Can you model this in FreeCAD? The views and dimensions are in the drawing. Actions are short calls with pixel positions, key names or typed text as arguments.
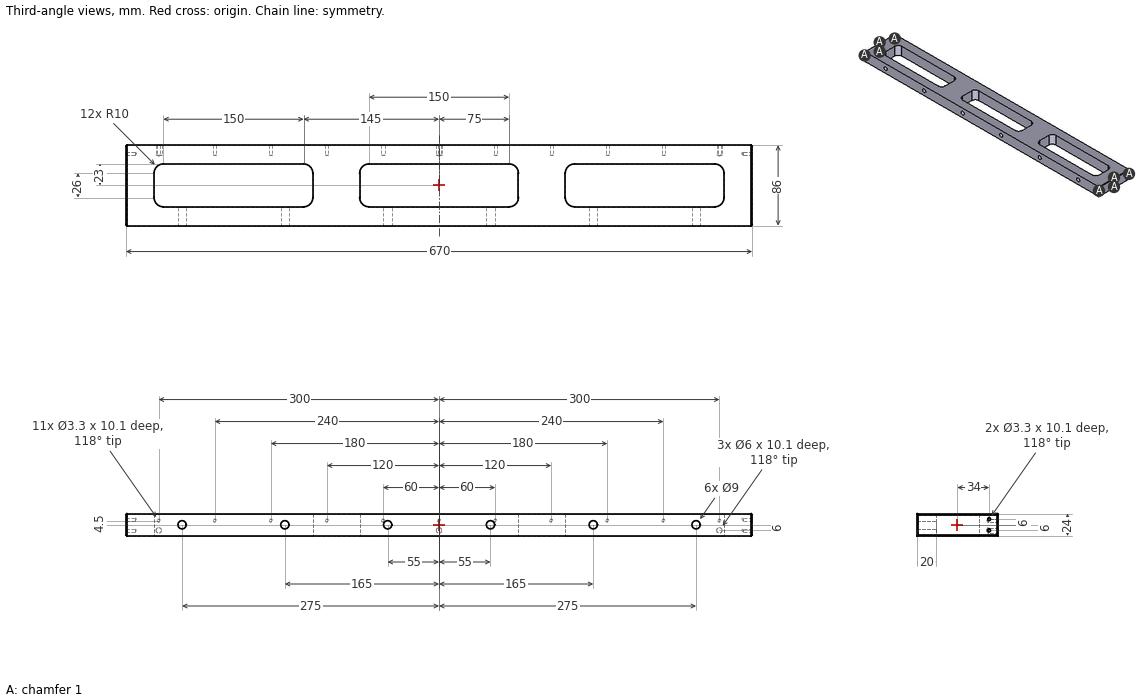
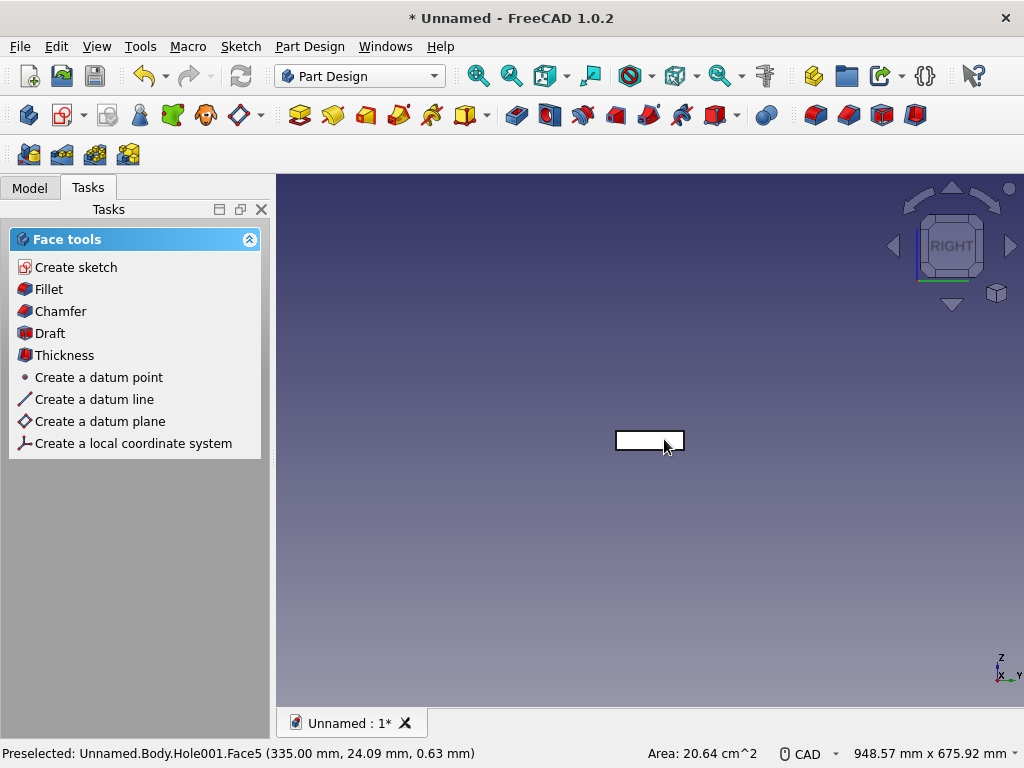
key(5)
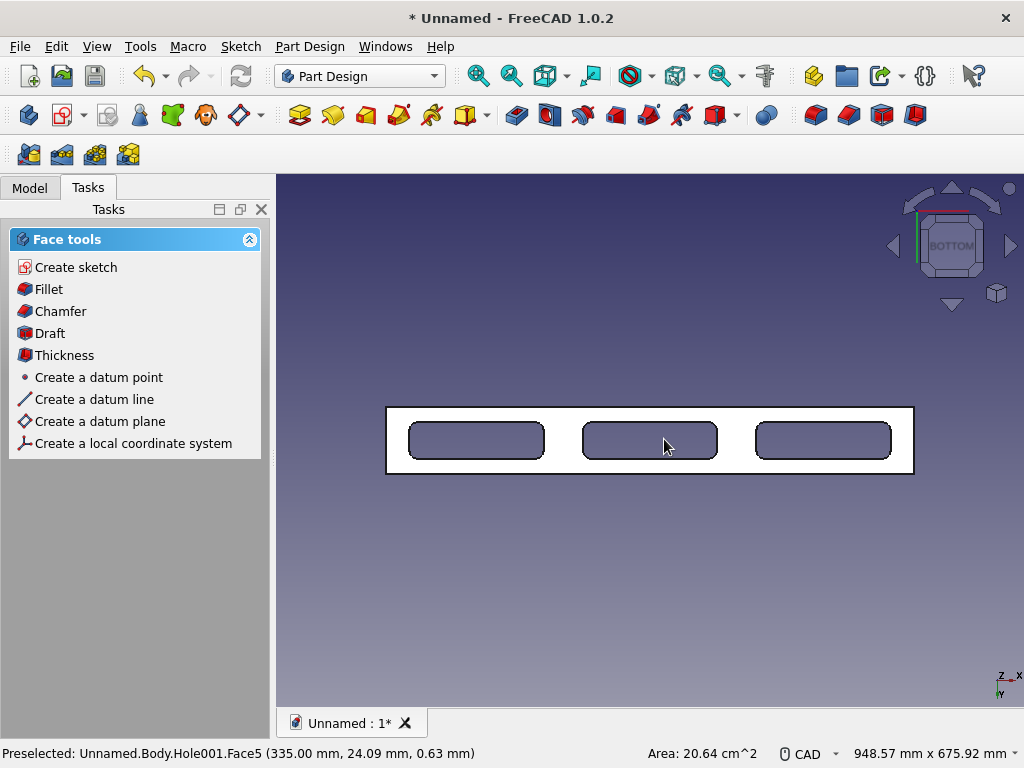
key(4)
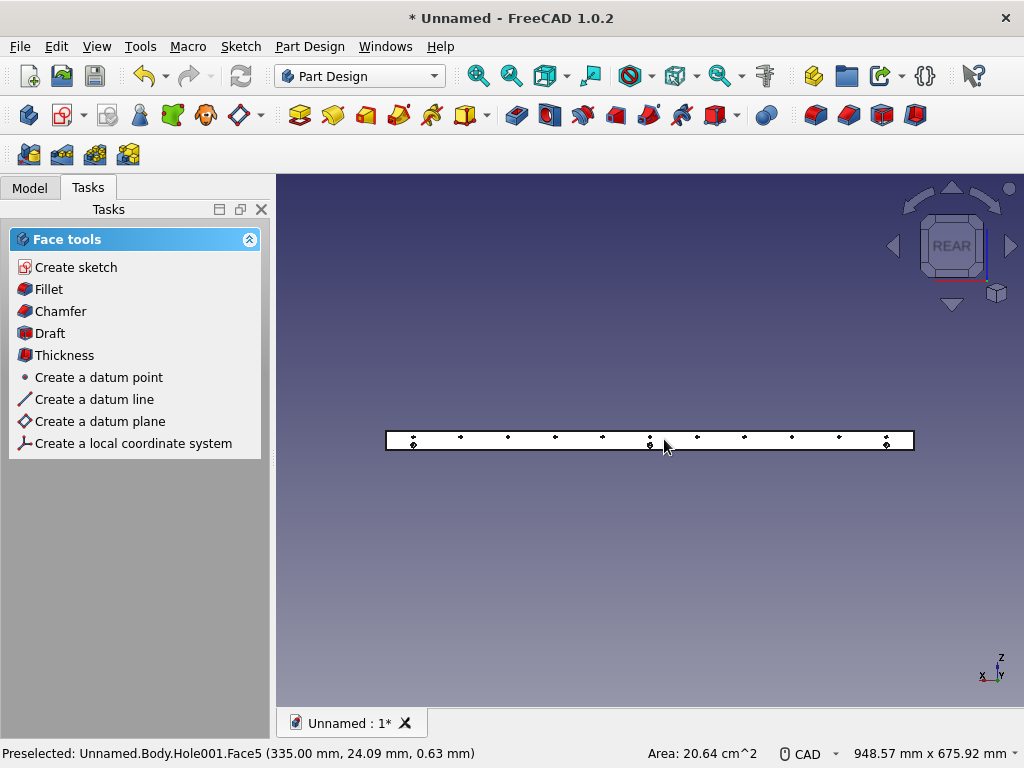
key(6)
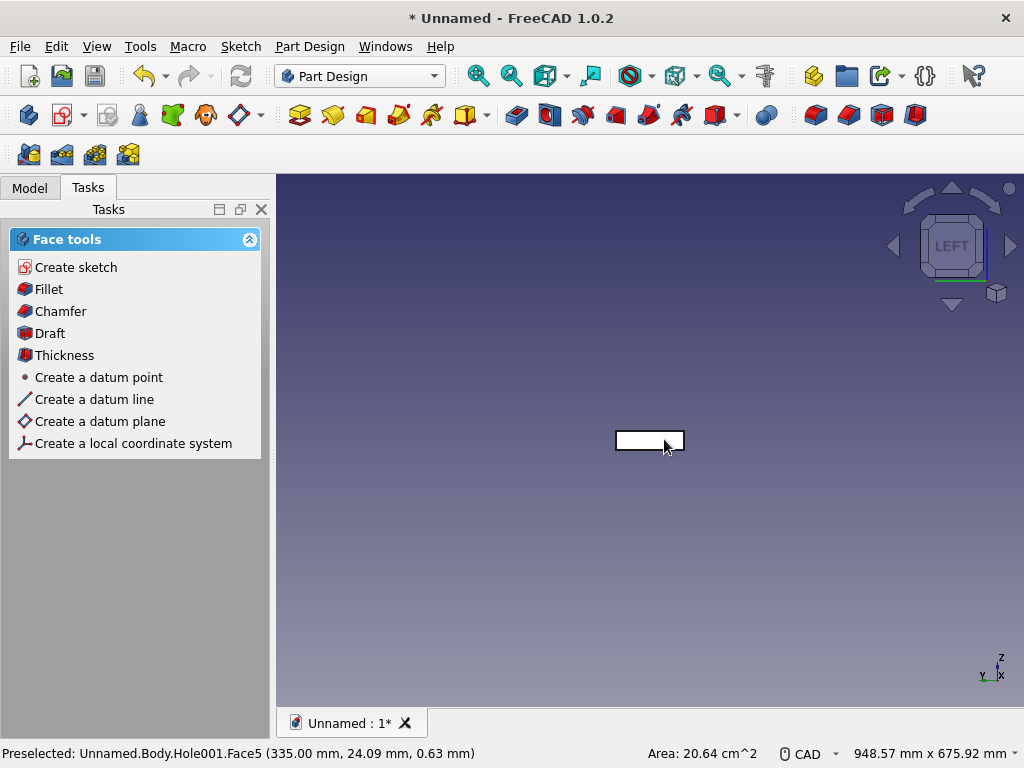
key(v)
key(f)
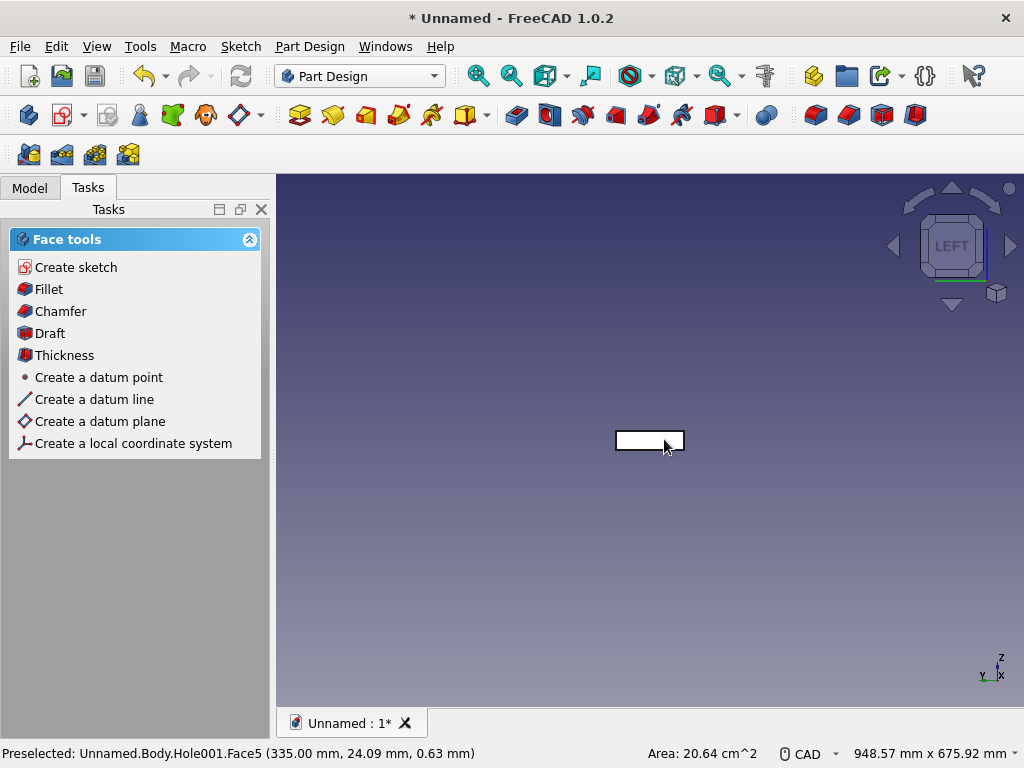
click(631, 439, ctrl)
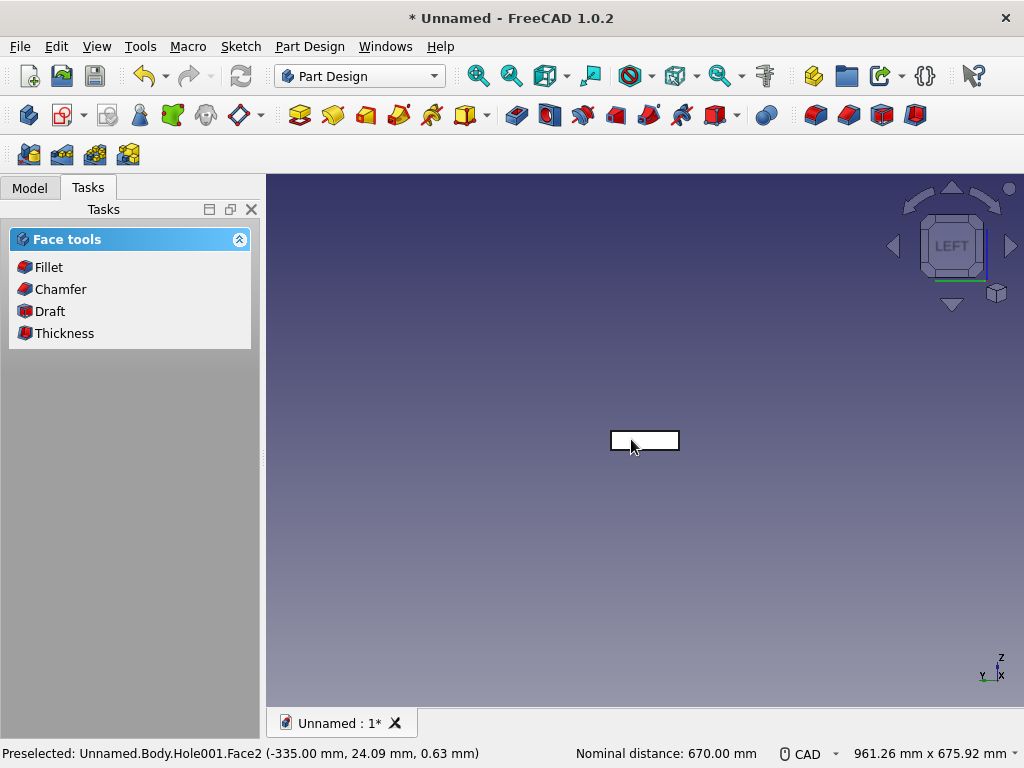
click(849, 116)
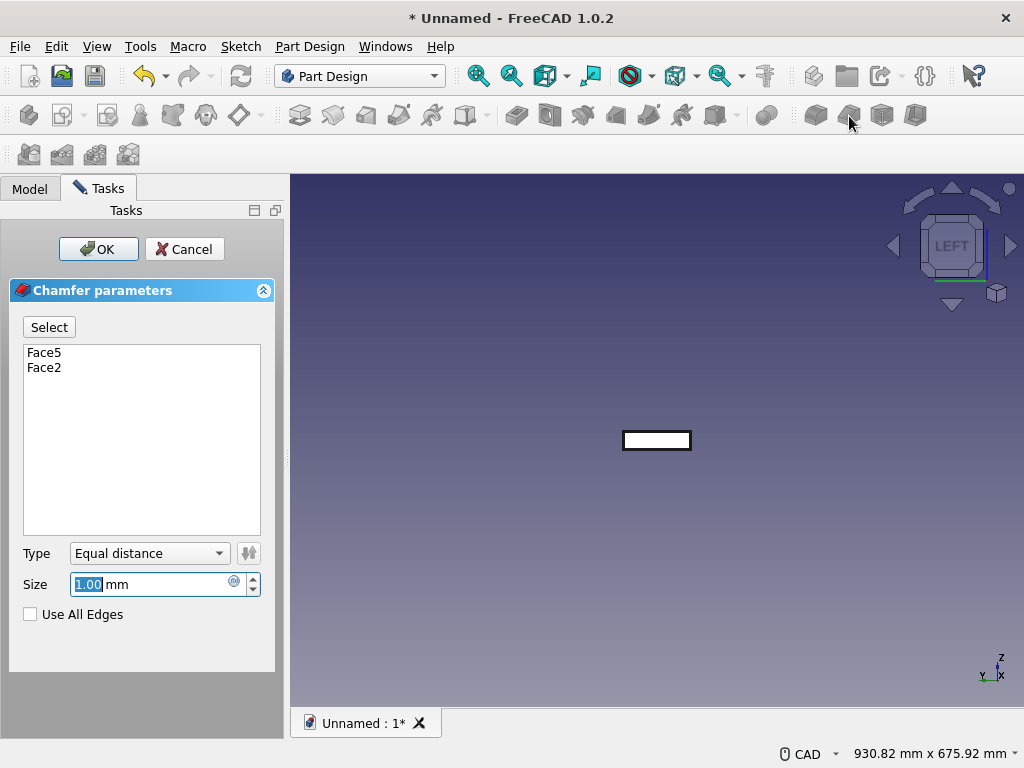
text(1)
key(Tab)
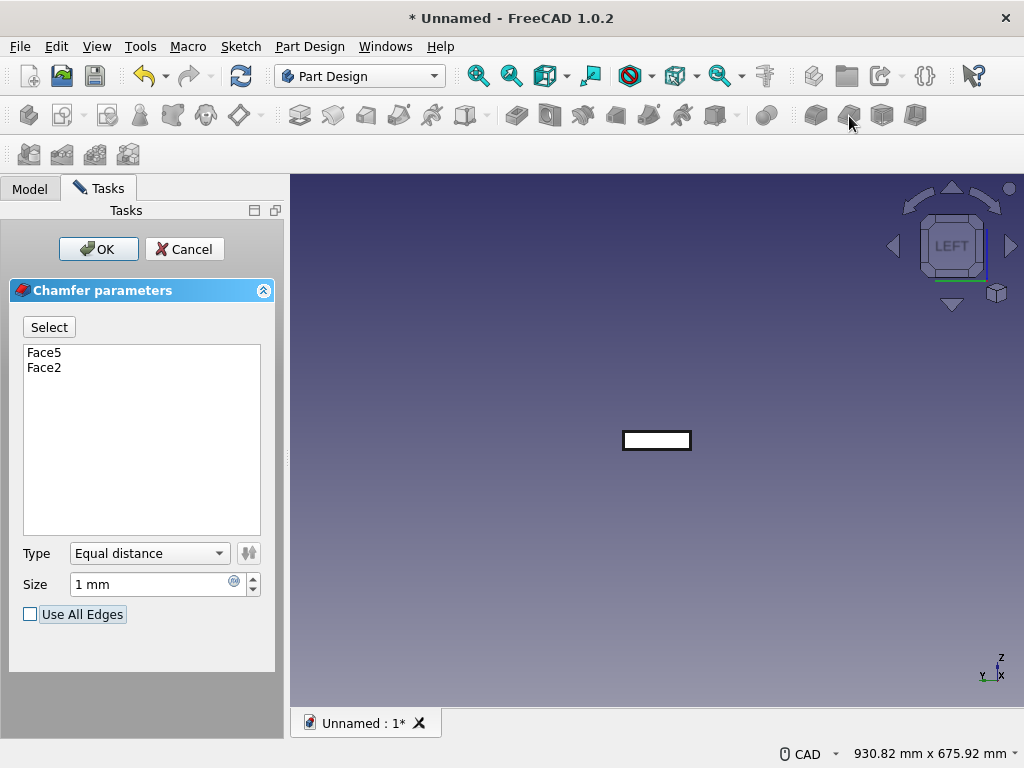
click(99, 249)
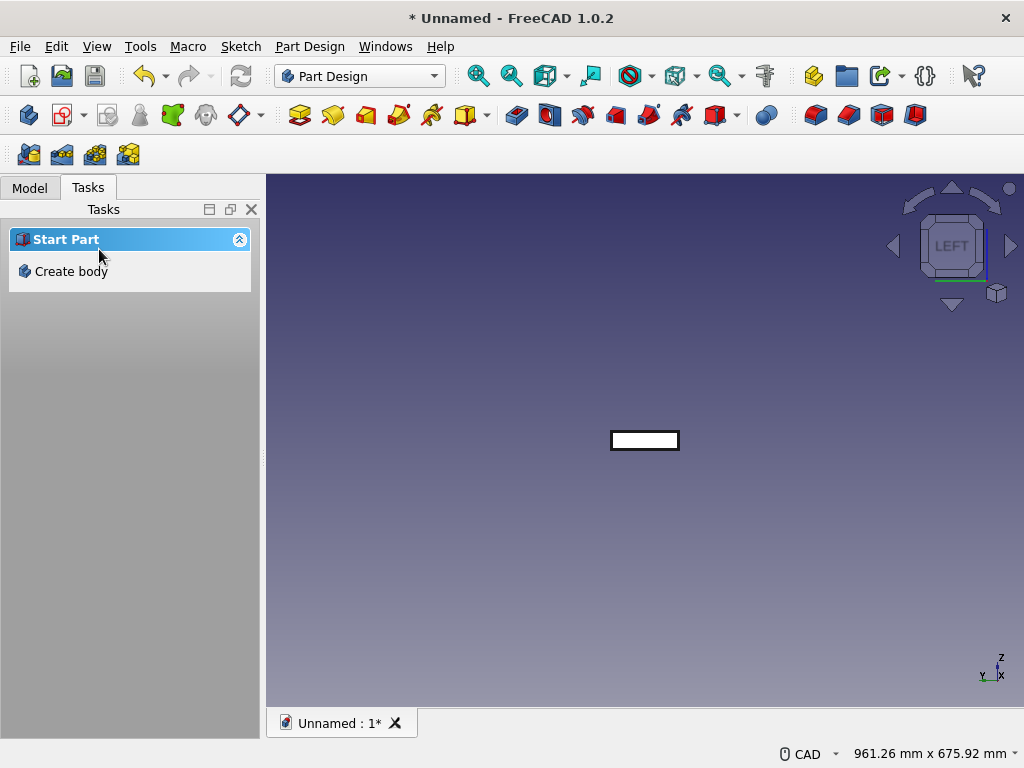
key(v)
key(f)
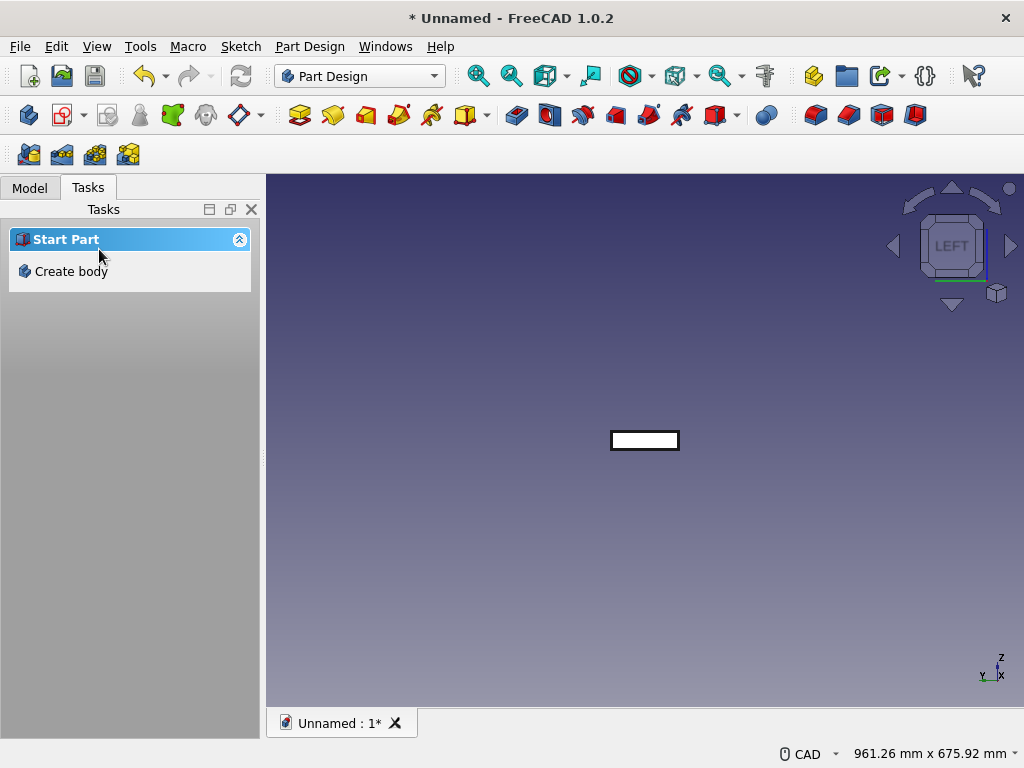
click(626, 439)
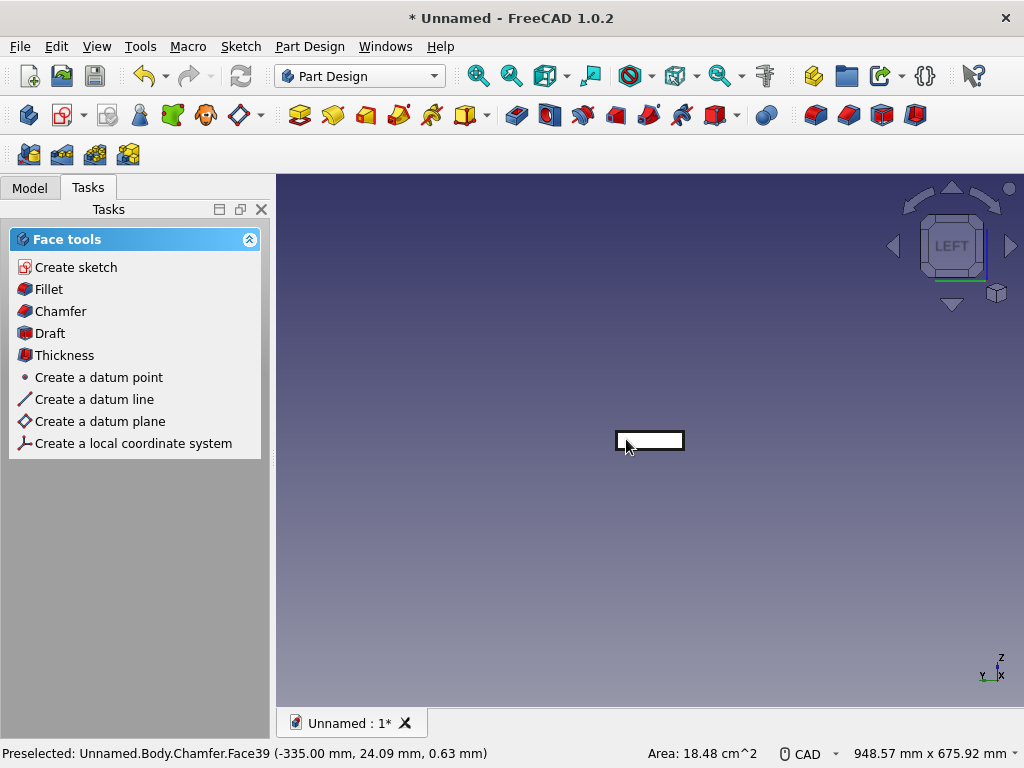
click(62, 116)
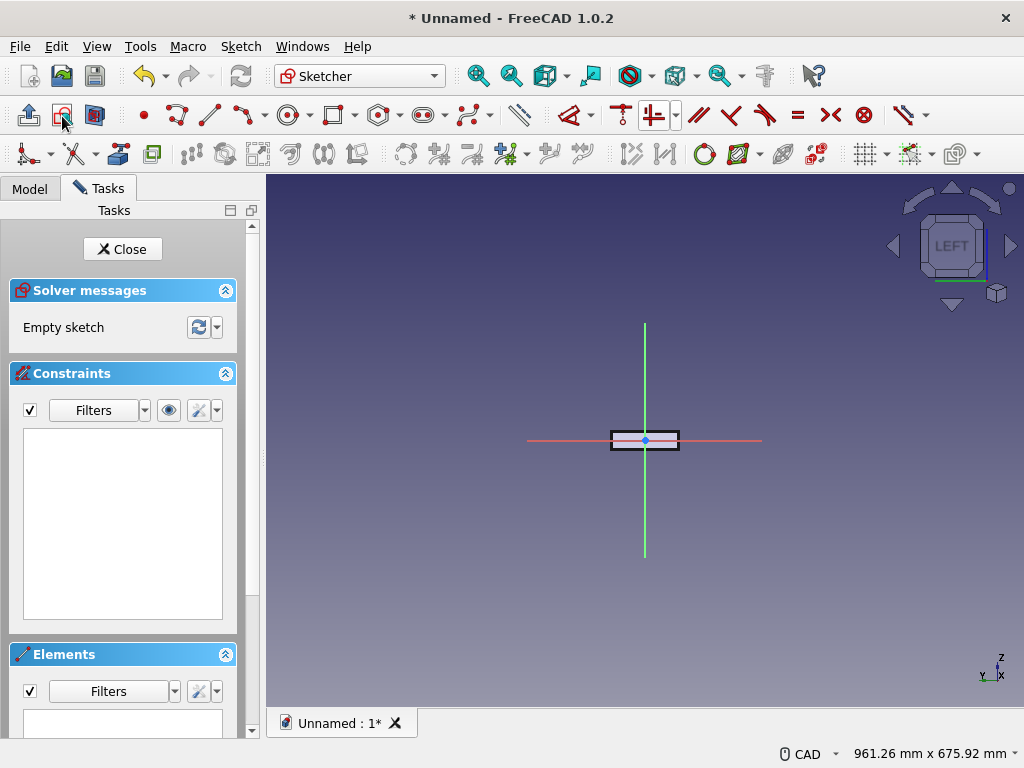
scroll(635, 440, up, 13)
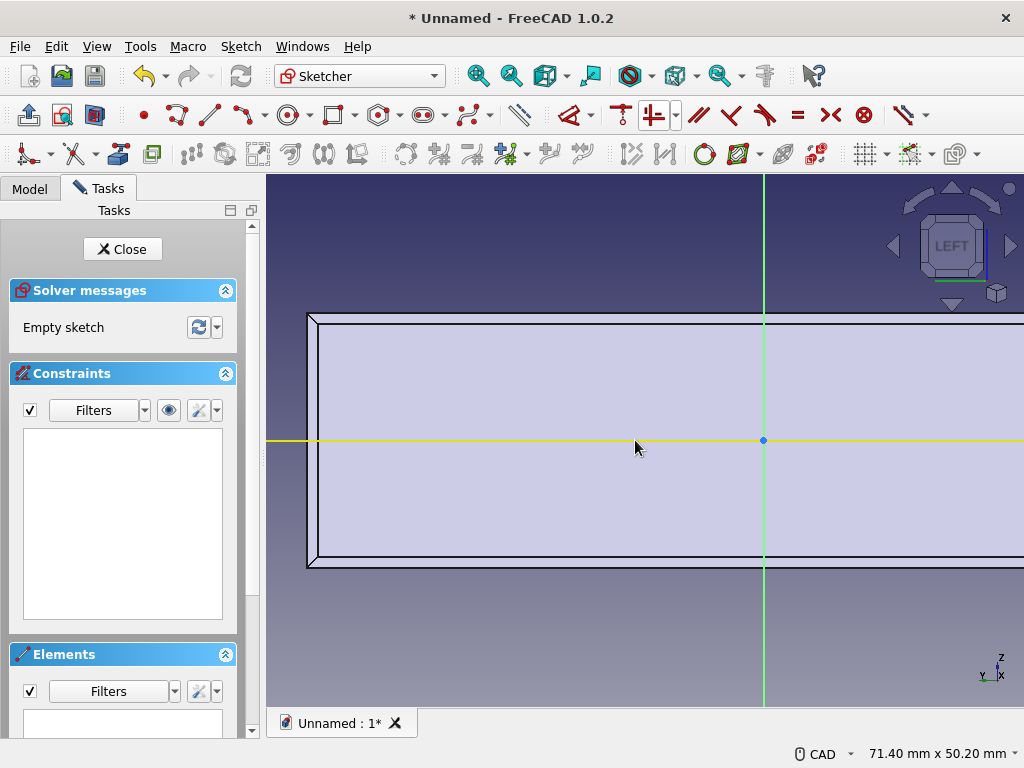
key(g)
key(c)